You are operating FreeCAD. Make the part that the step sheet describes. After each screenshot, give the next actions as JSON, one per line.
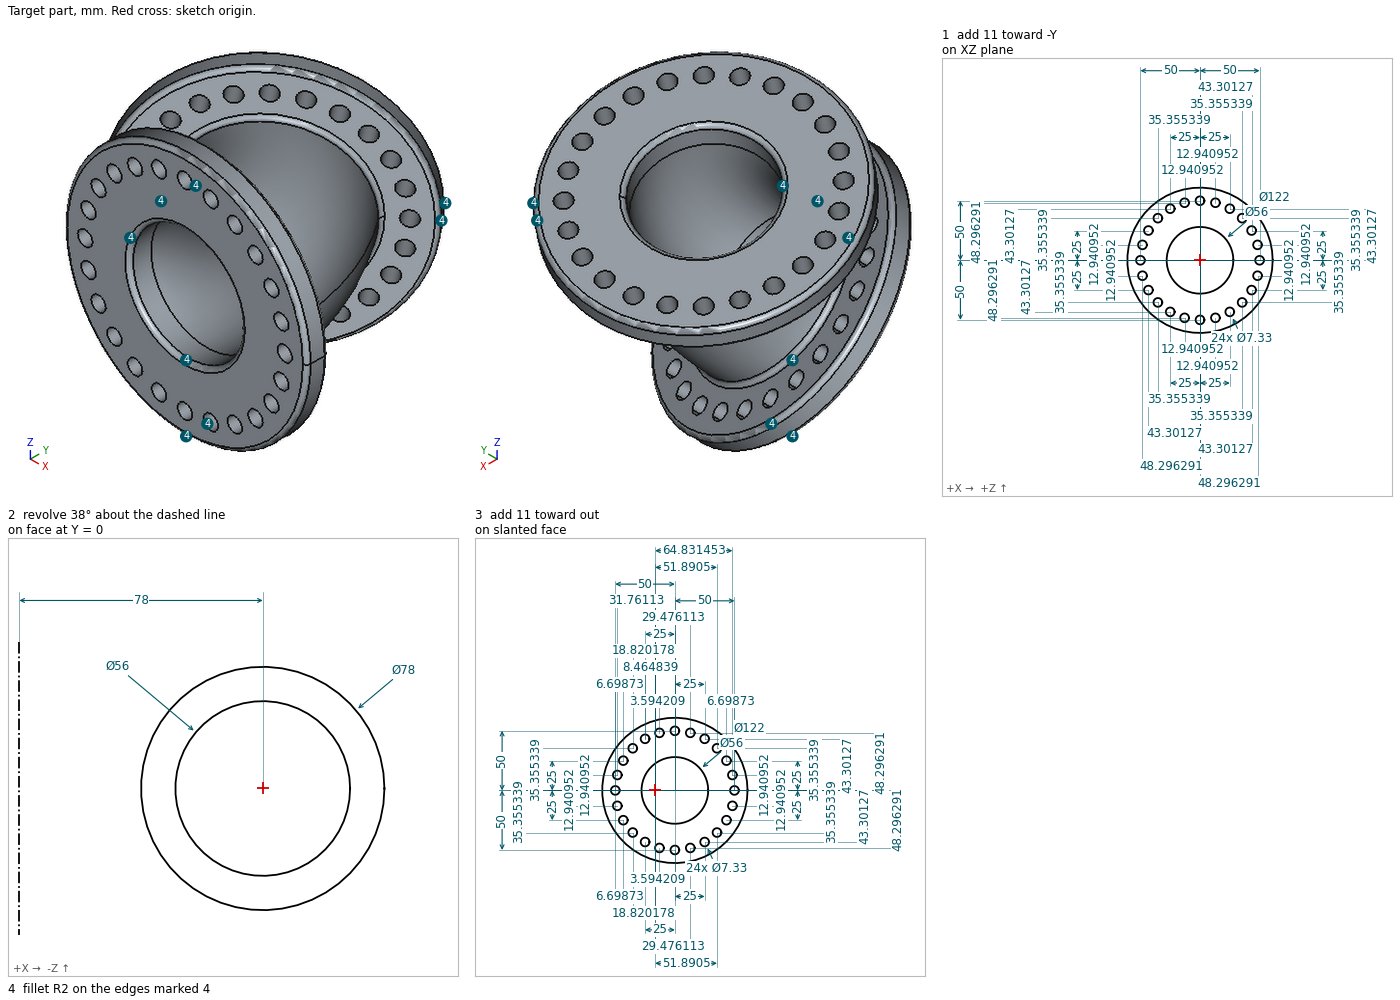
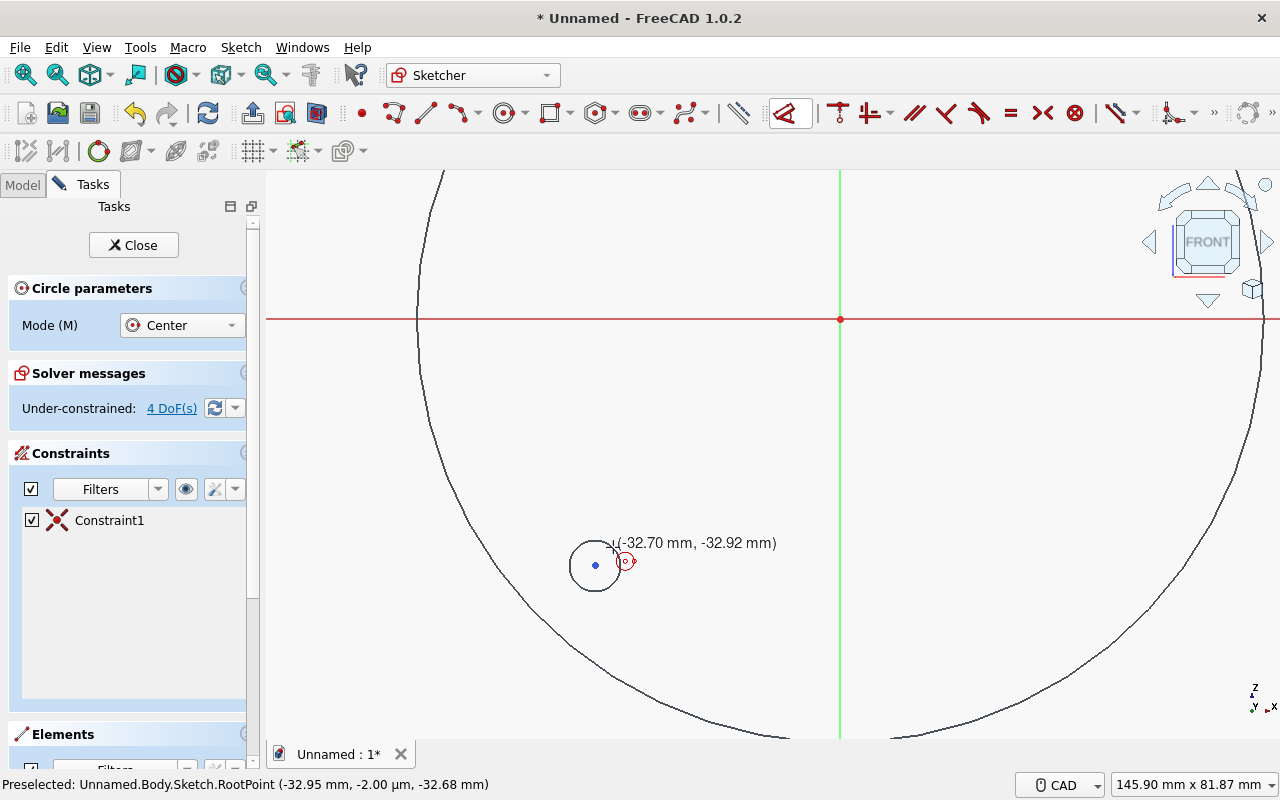
{"action": "left_click", "coordinate": [539, 493]}
{"action": "left_click", "coordinate": [557, 475]}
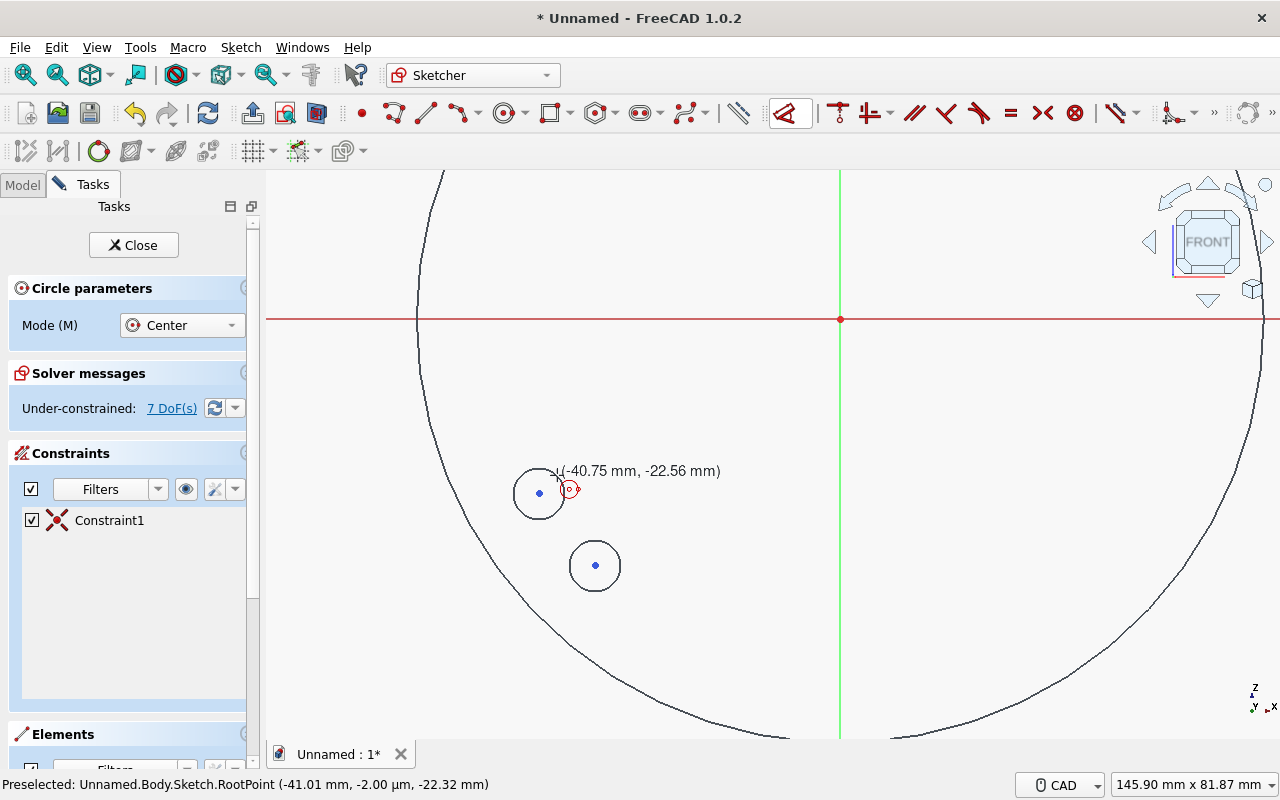
{"action": "left_click", "coordinate": [505, 409]}
{"action": "left_click", "coordinate": [523, 391]}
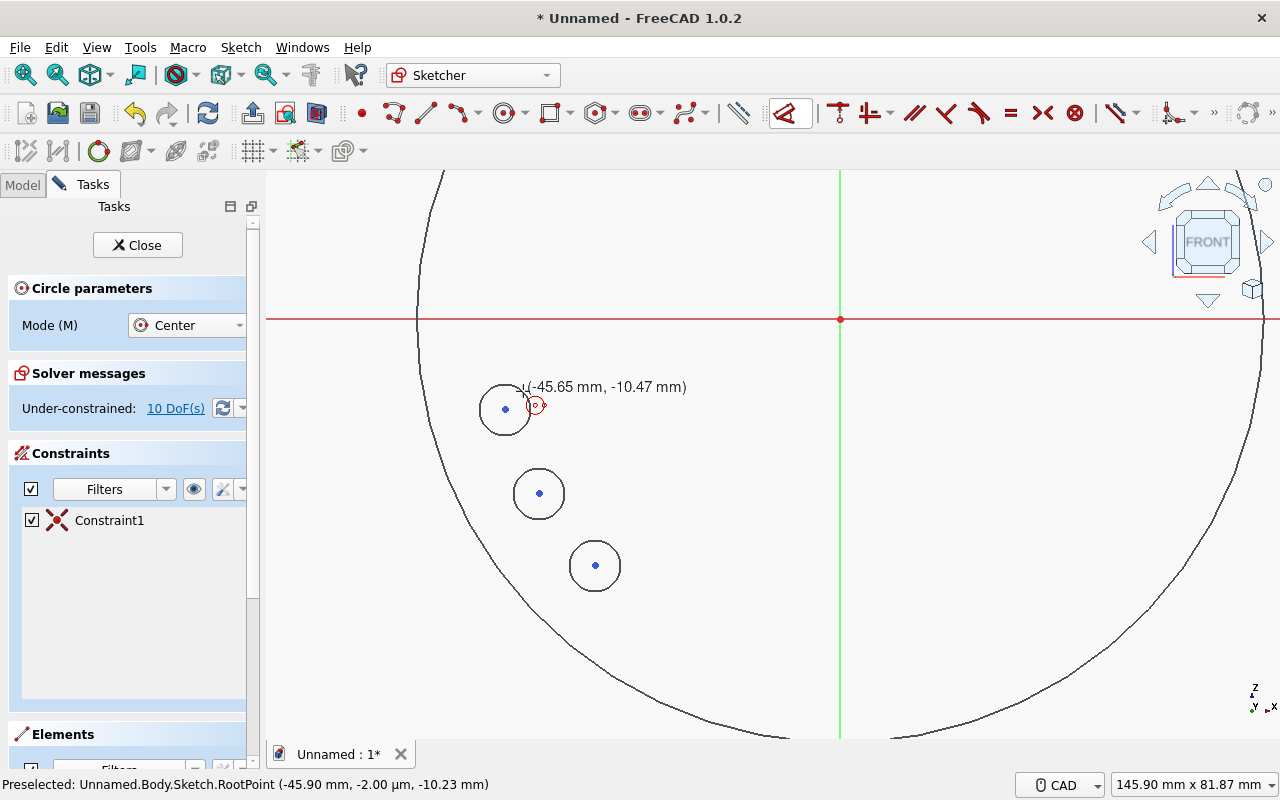
{"action": "left_click", "coordinate": [666, 620]}
{"action": "left_click", "coordinate": [684, 602]}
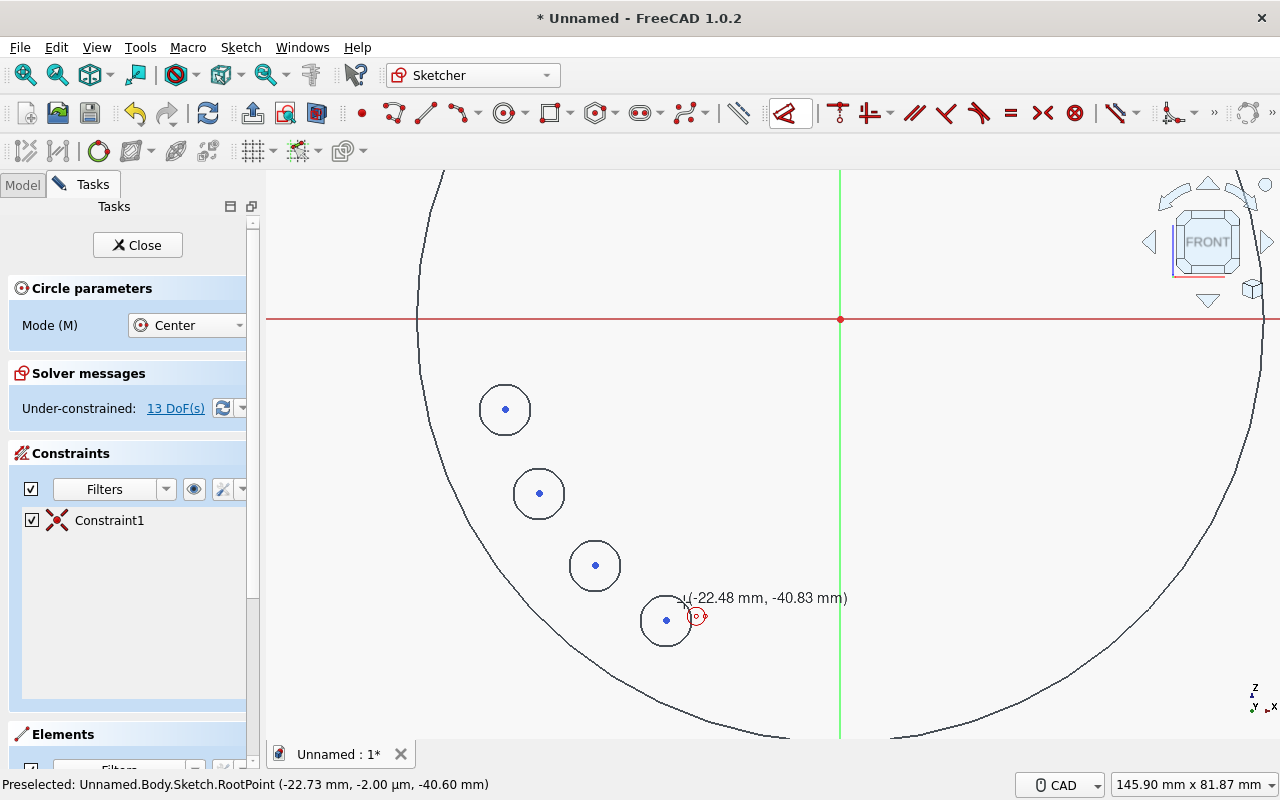
{"action": "left_click", "coordinate": [750, 655]}
{"action": "left_click", "coordinate": [768, 637]}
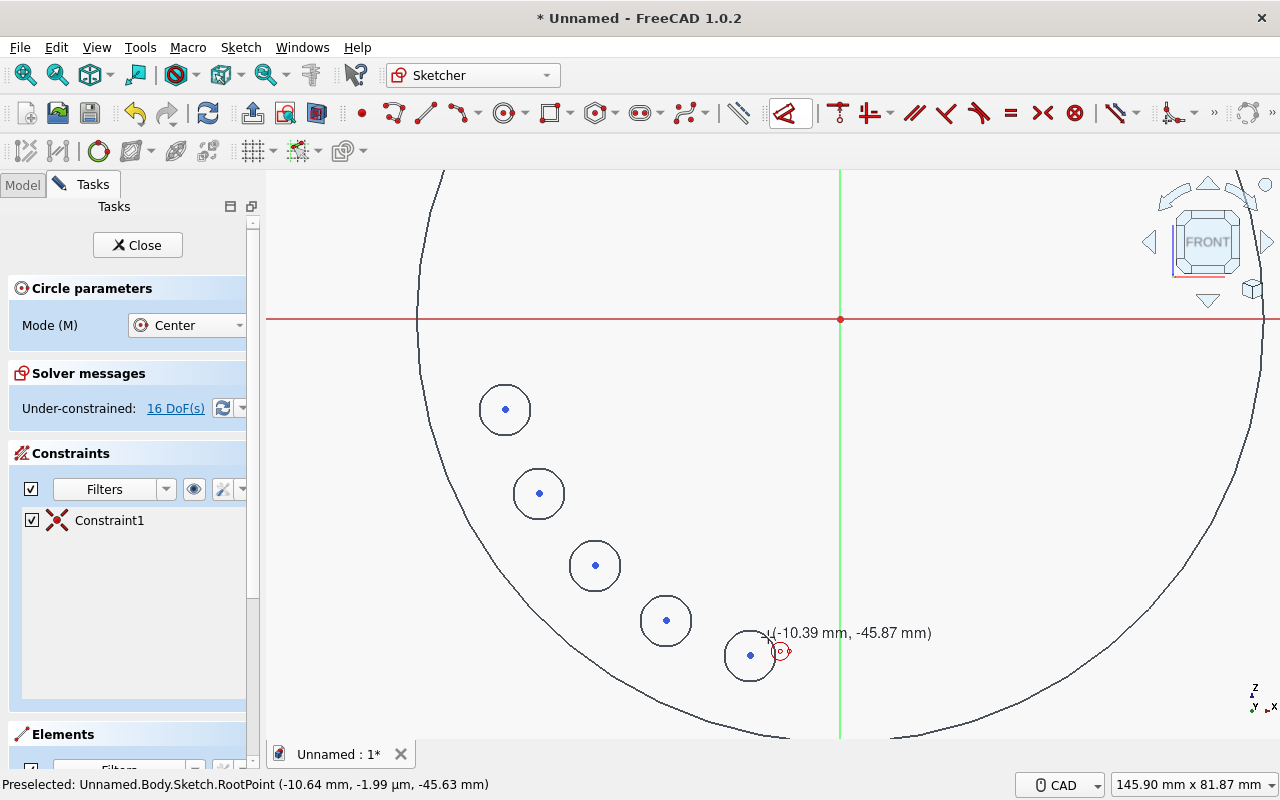
{"action": "left_click", "coordinate": [840, 667]}
{"action": "left_click", "coordinate": [858, 649]}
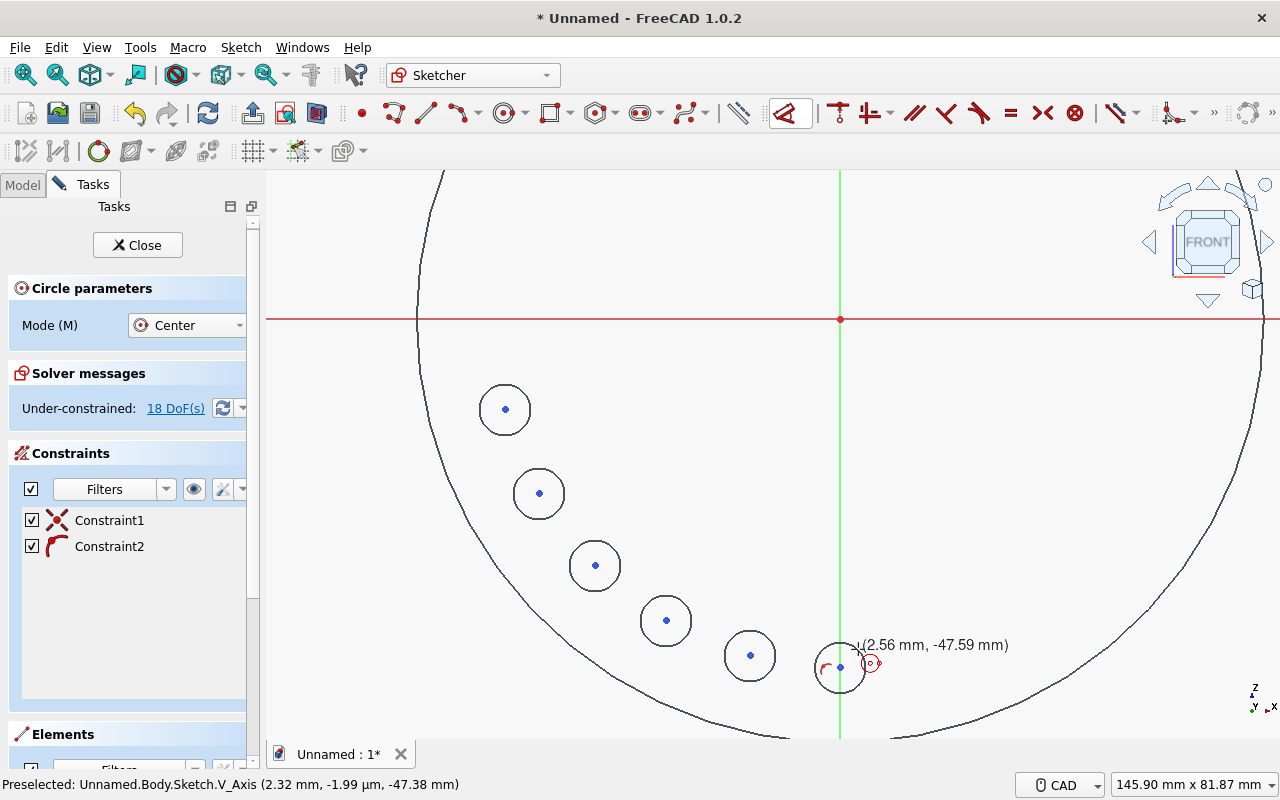
{"action": "left_click", "coordinate": [840, 319]}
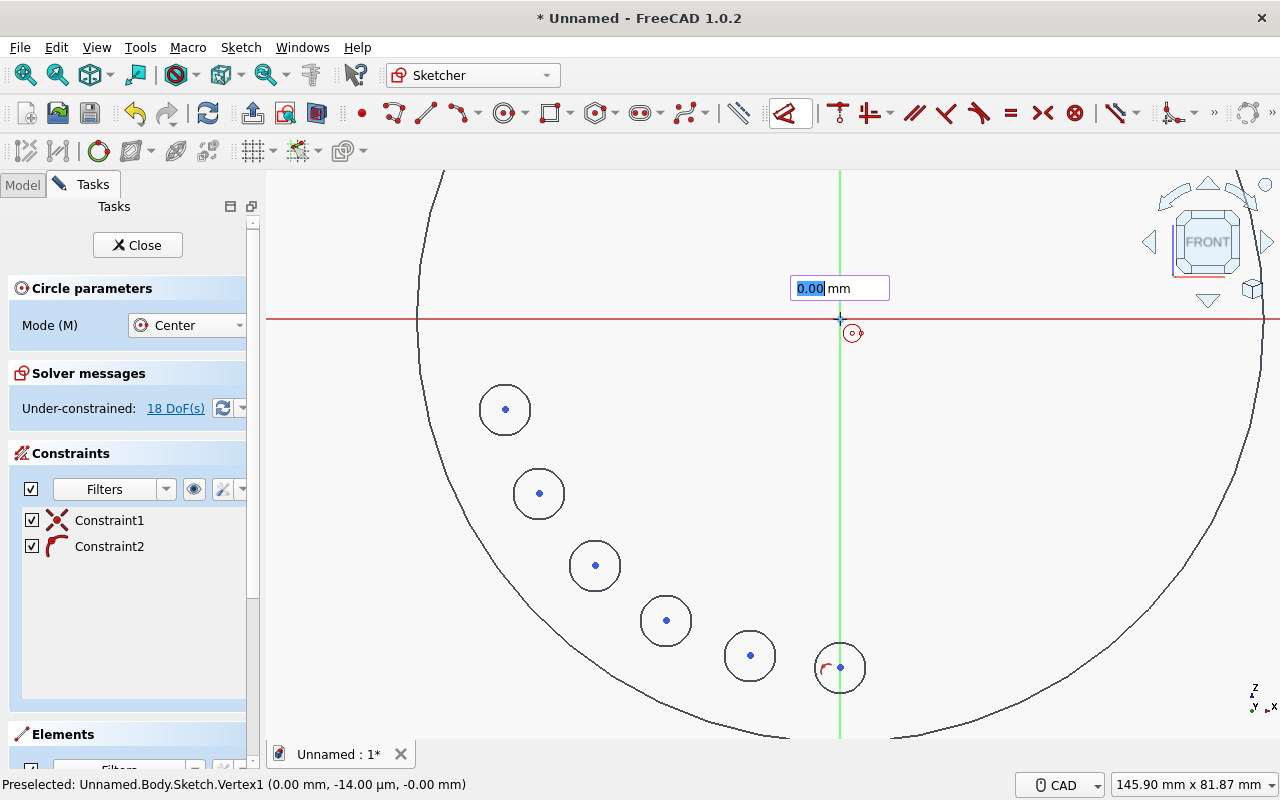
{"action": "scroll", "coordinate": [594, 565], "scroll_direction": "down", "scroll_amount": 4}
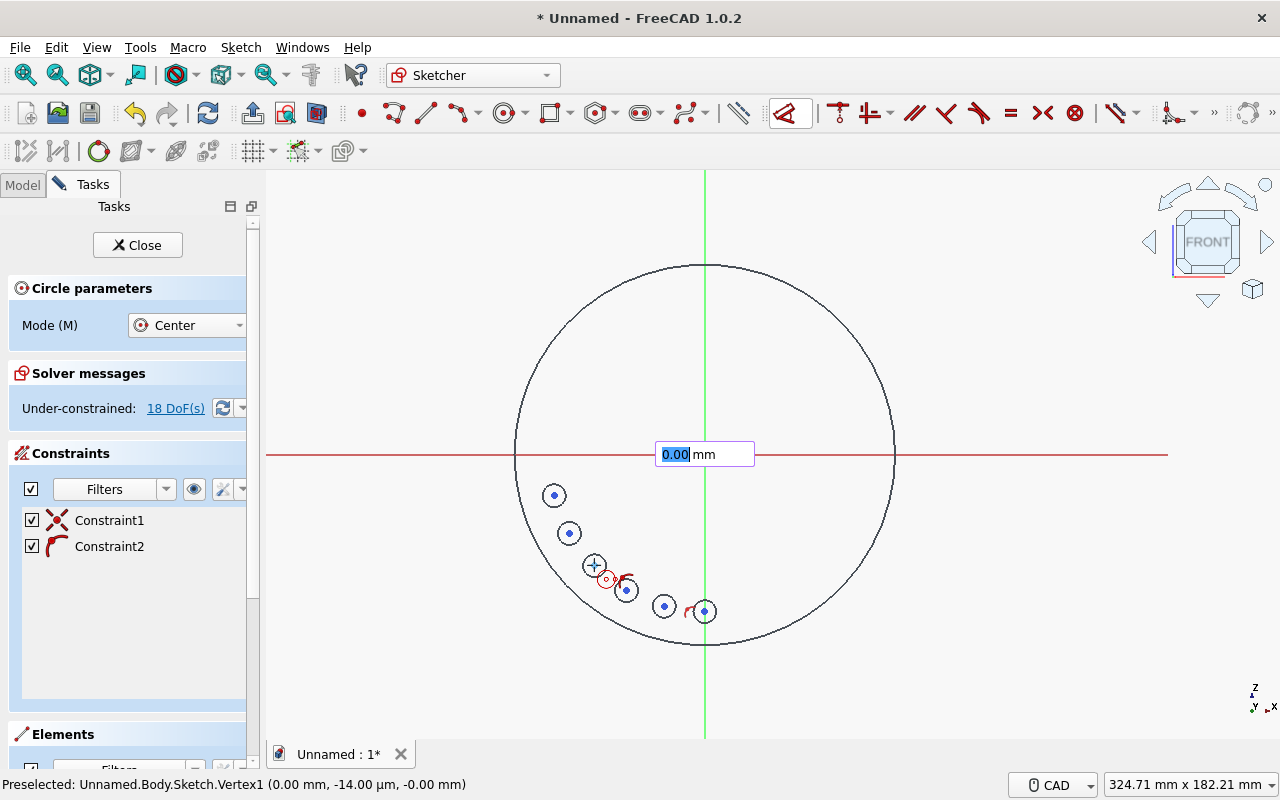
{"action": "left_click", "coordinate": [767, 393]}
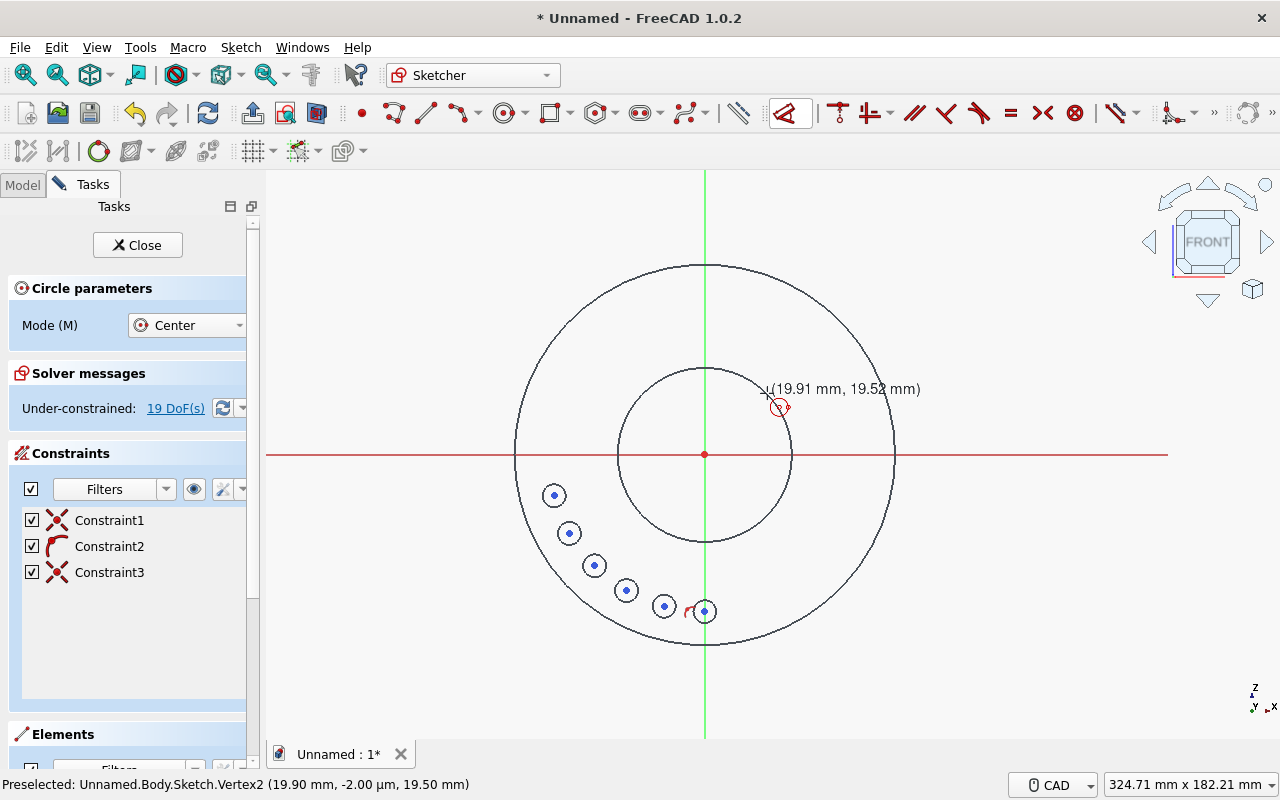
{"action": "scroll", "coordinate": [549, 455], "scroll_direction": "up", "scroll_amount": 4}